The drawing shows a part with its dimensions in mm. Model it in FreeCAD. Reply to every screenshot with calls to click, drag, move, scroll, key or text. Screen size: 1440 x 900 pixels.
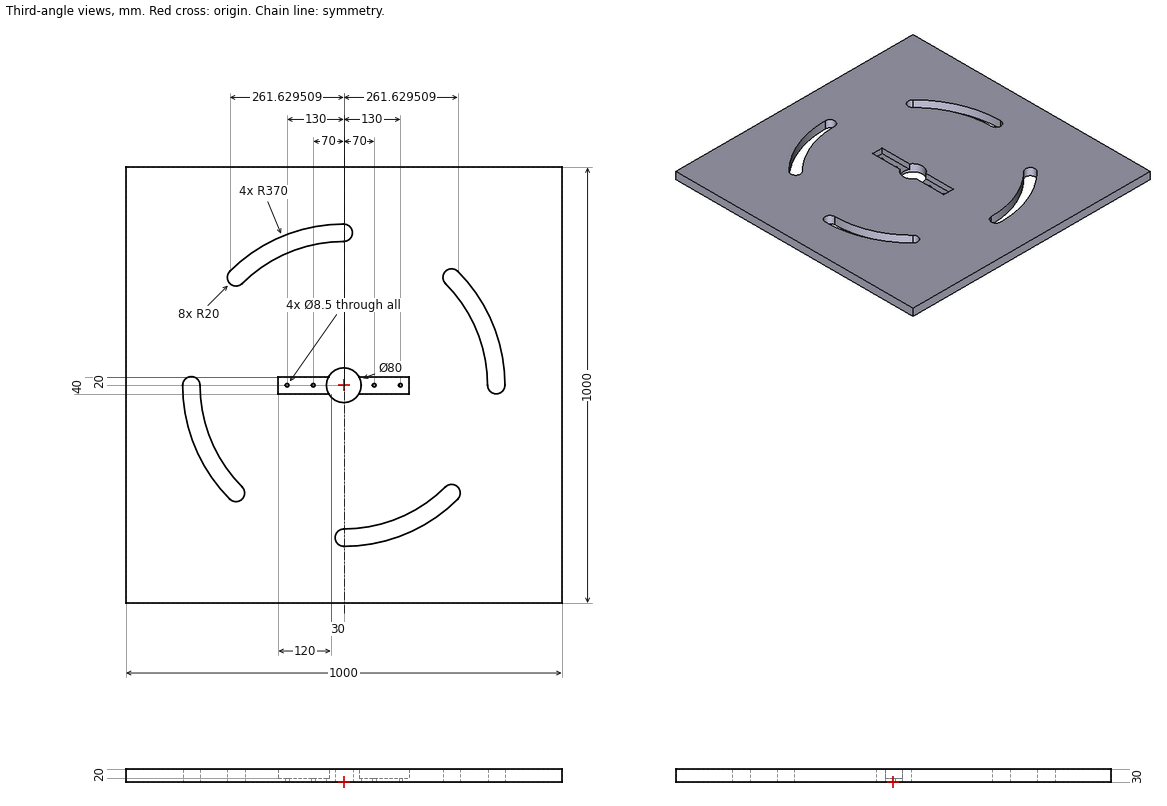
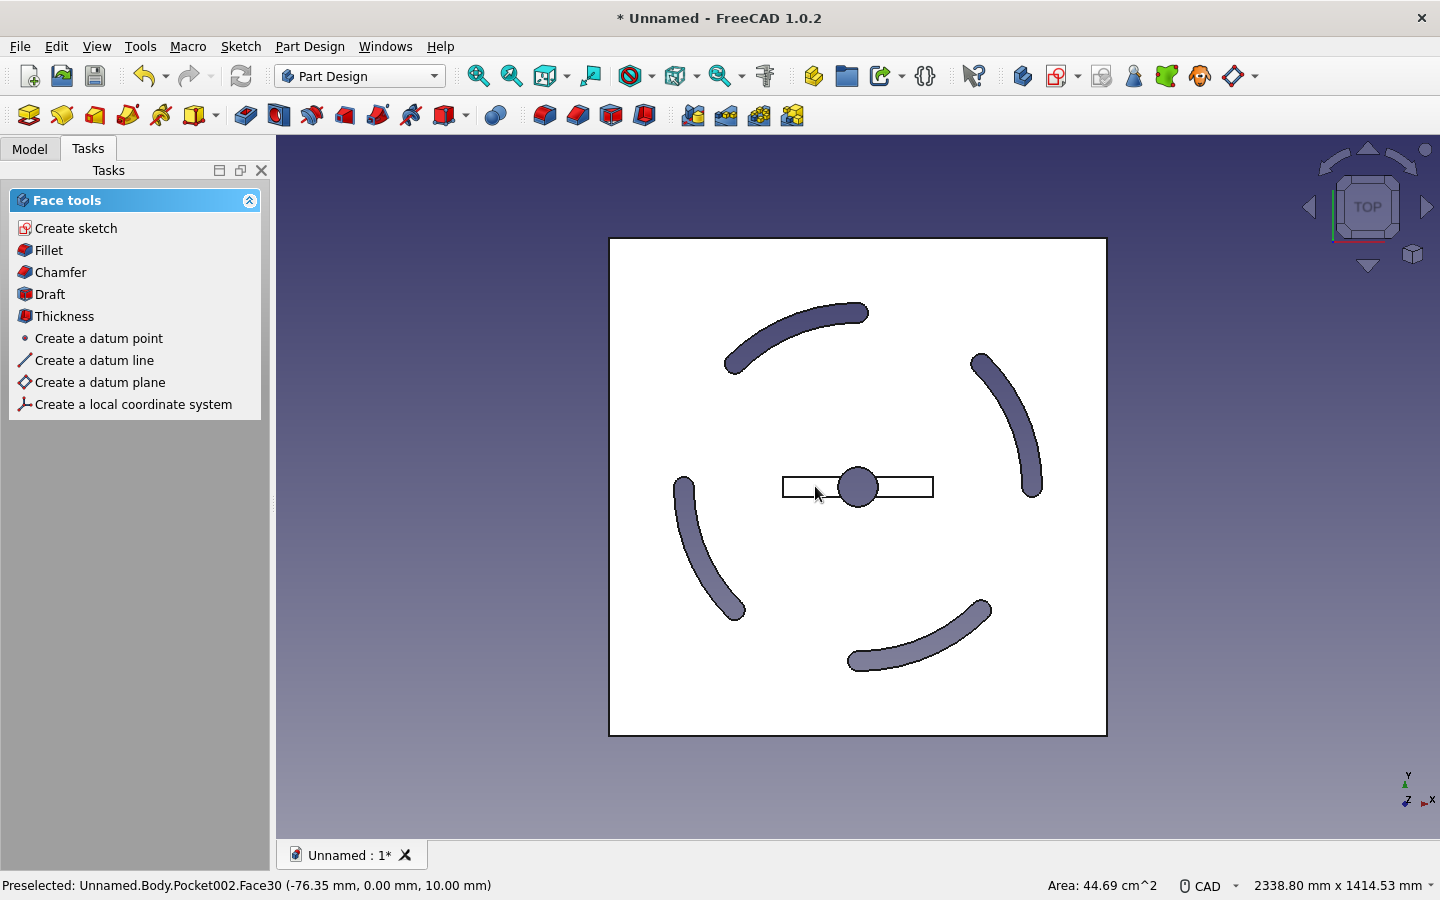
click(1056, 76)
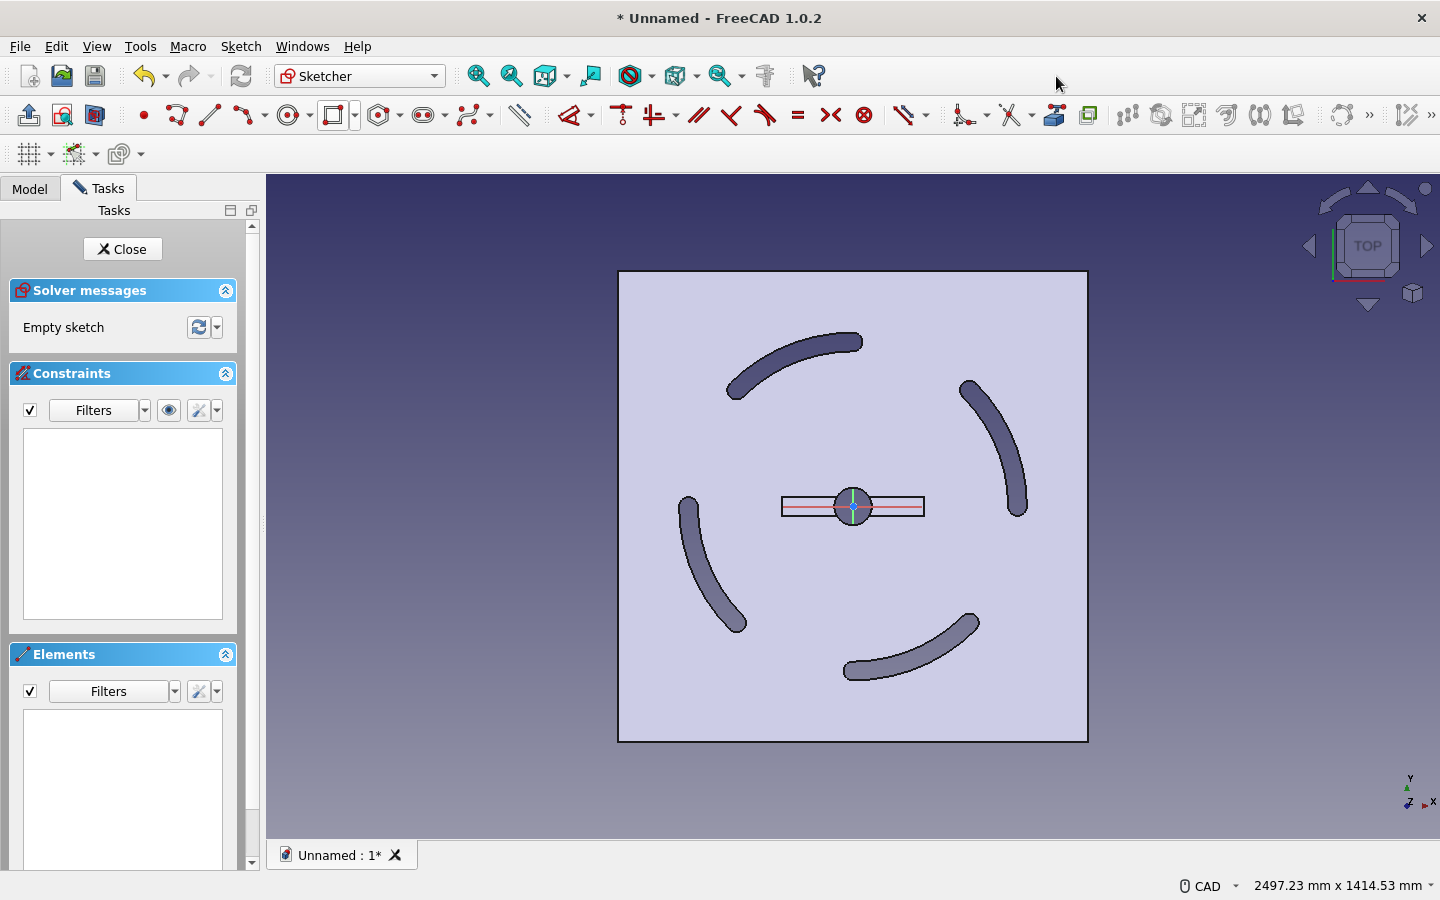
click(95, 116)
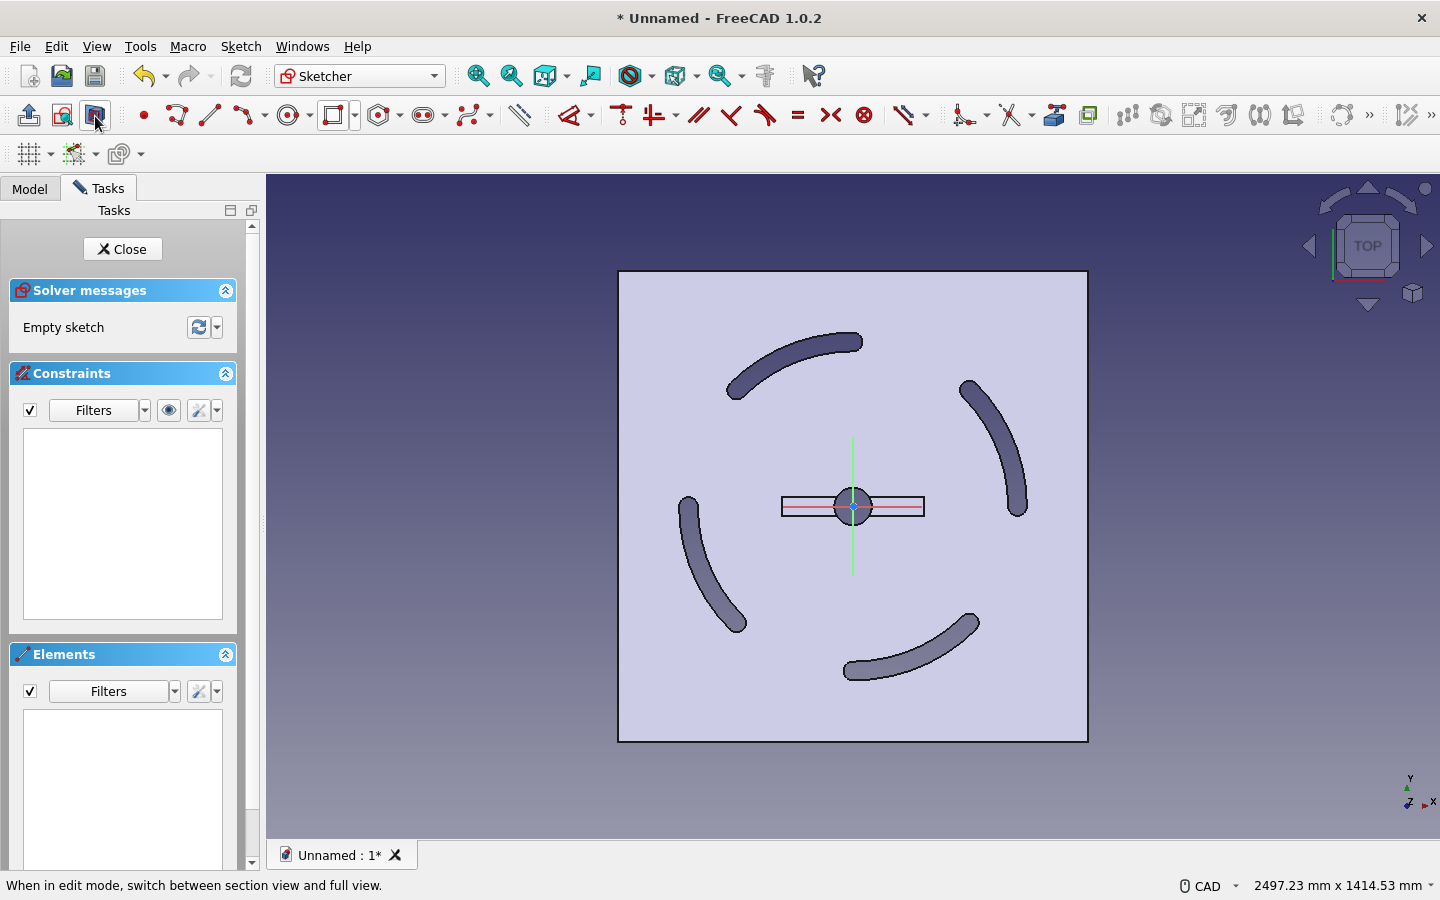
scroll(867, 506, up, 9)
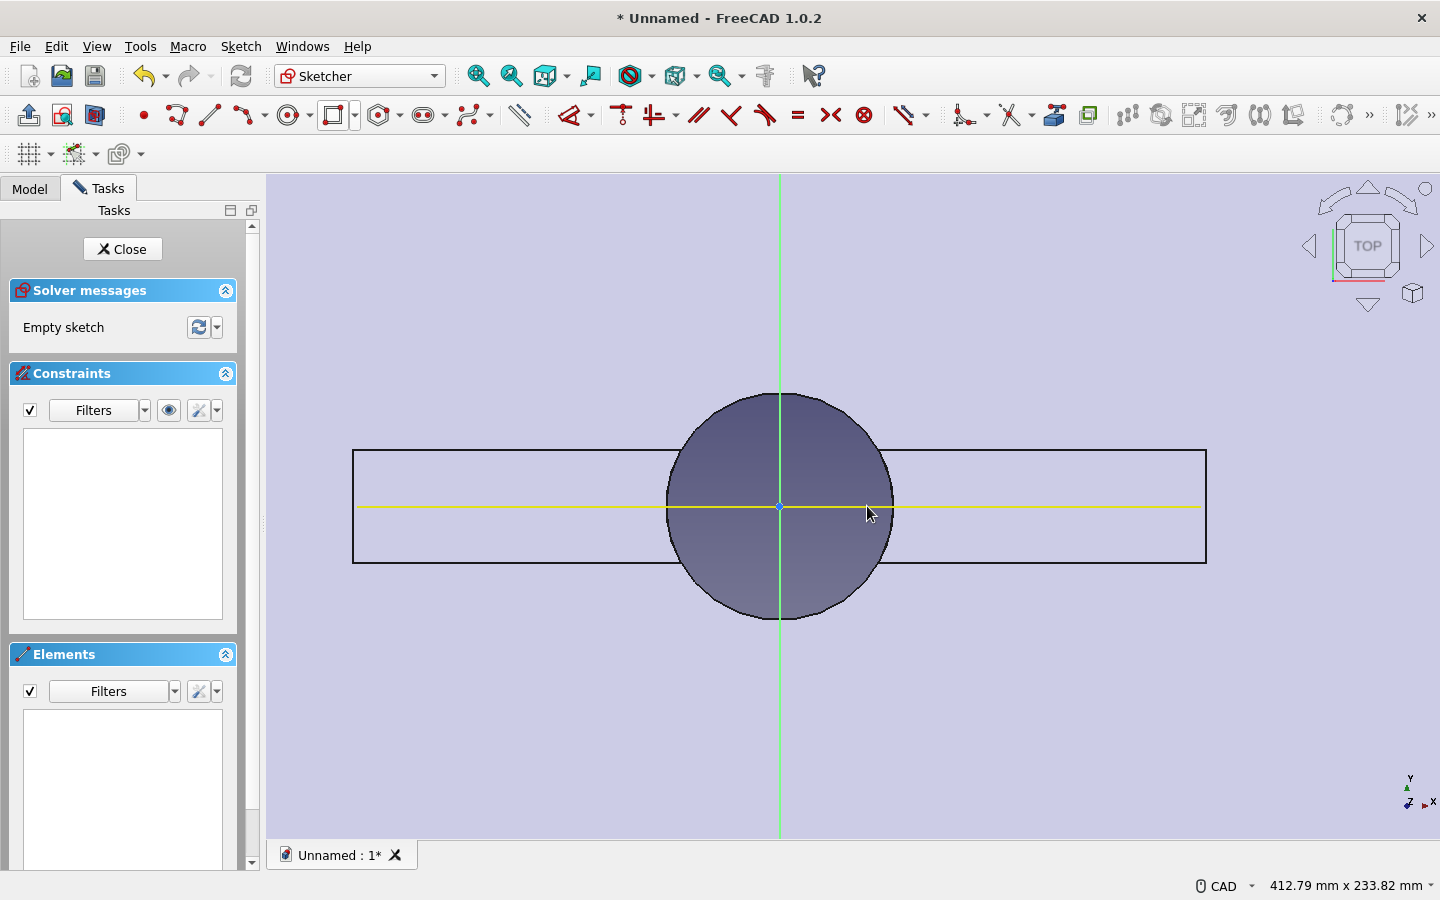
click(288, 116)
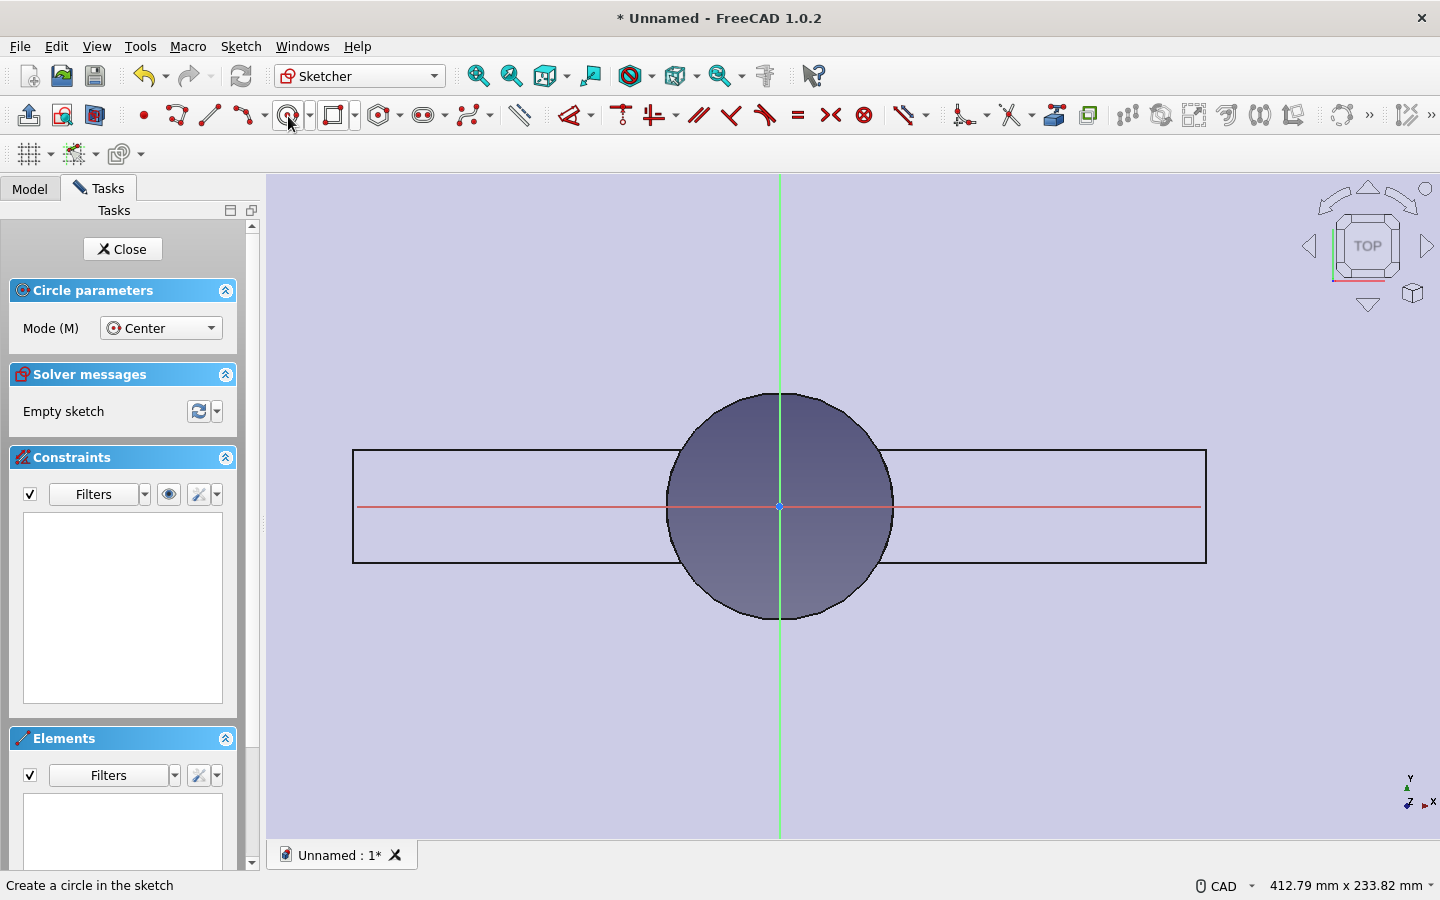
scroll(410, 506, up, 4)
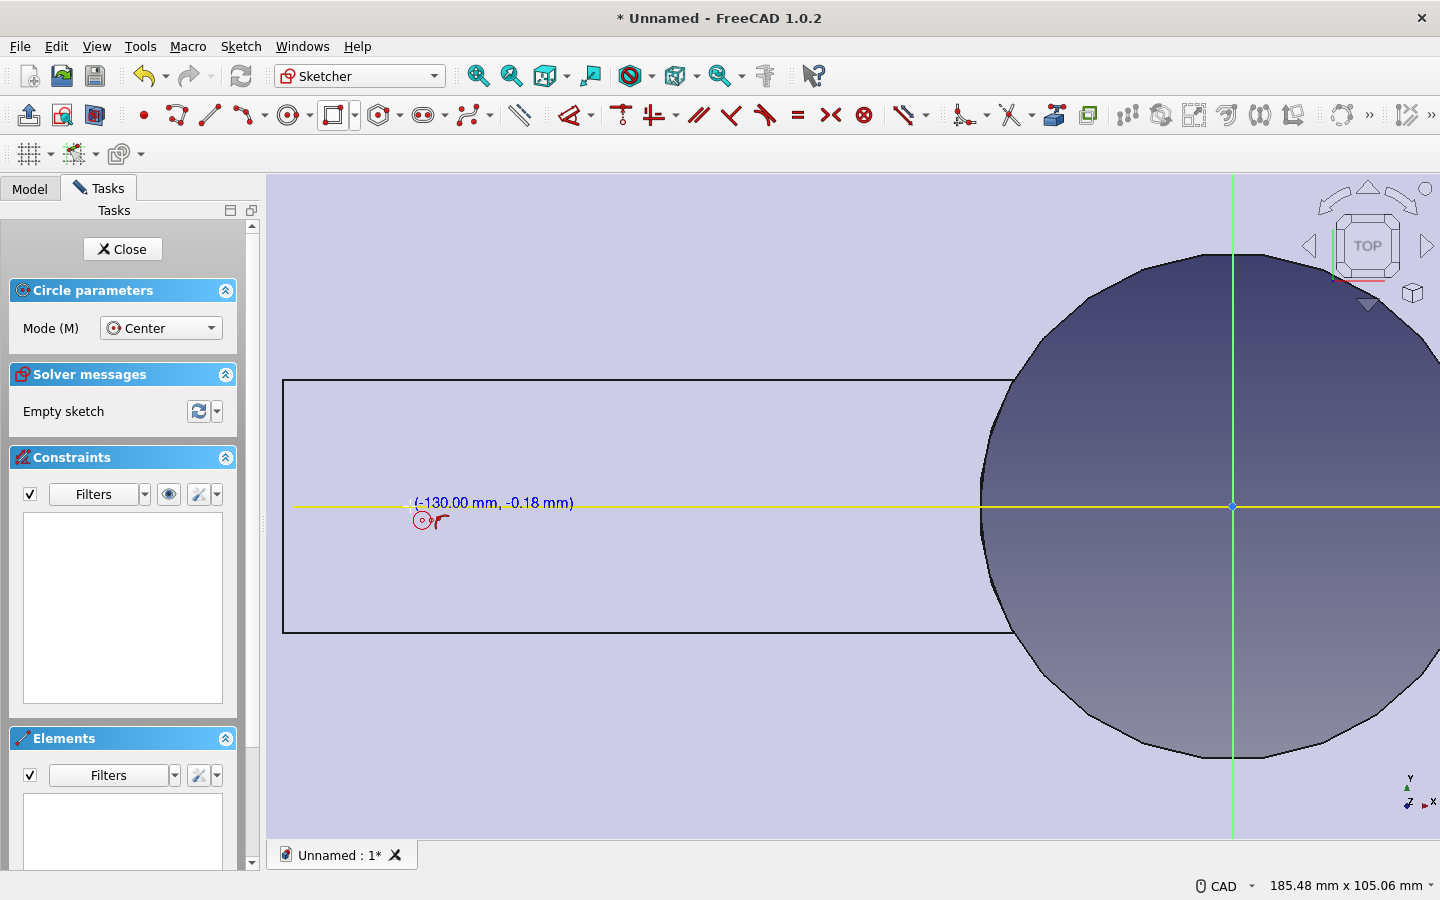
click(410, 506)
click(429, 487)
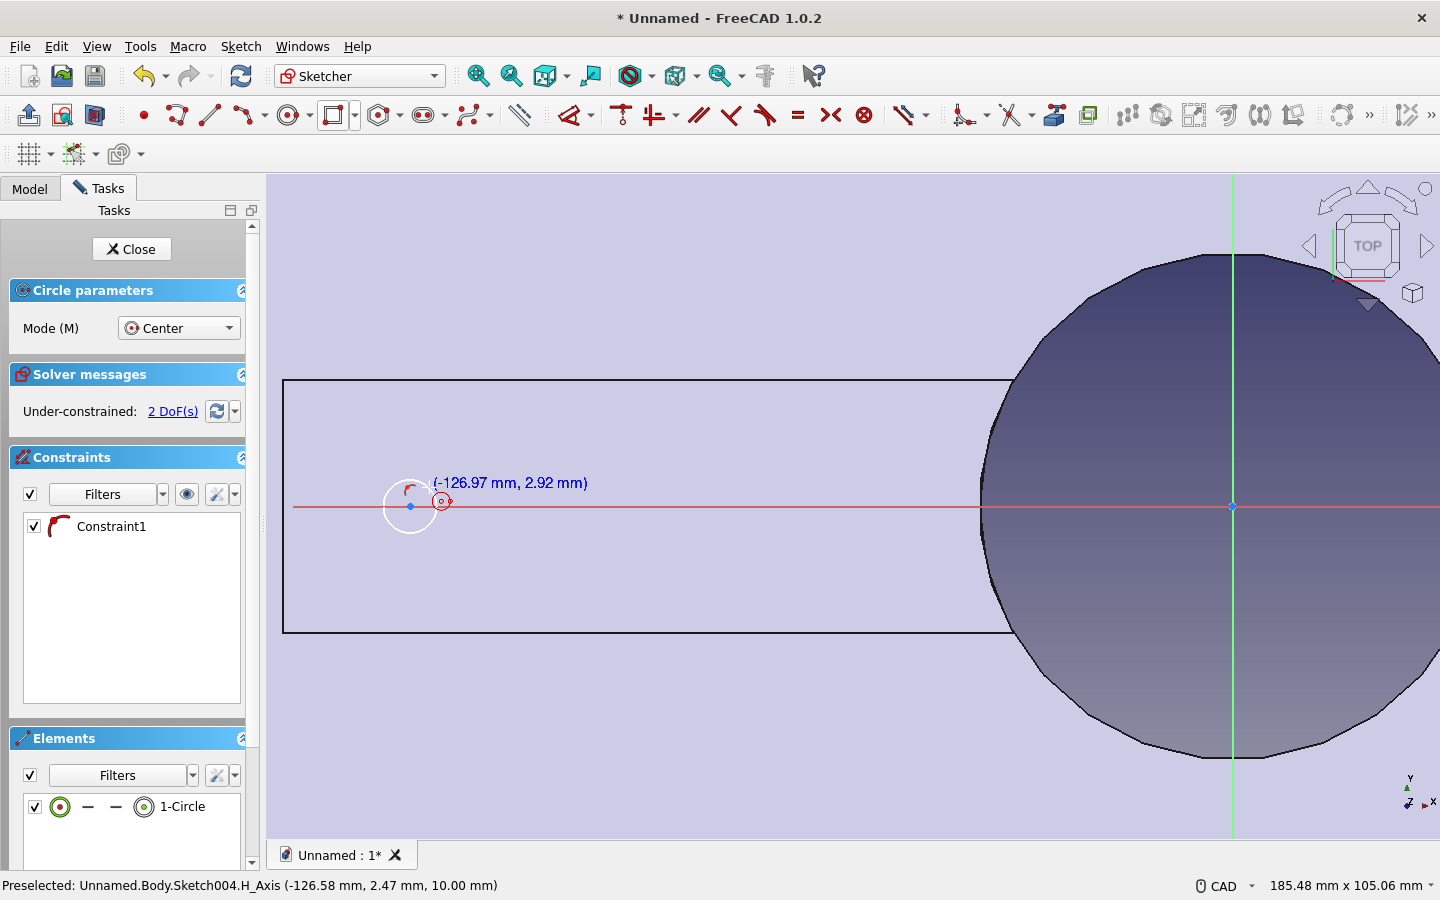
click(790, 506)
click(809, 487)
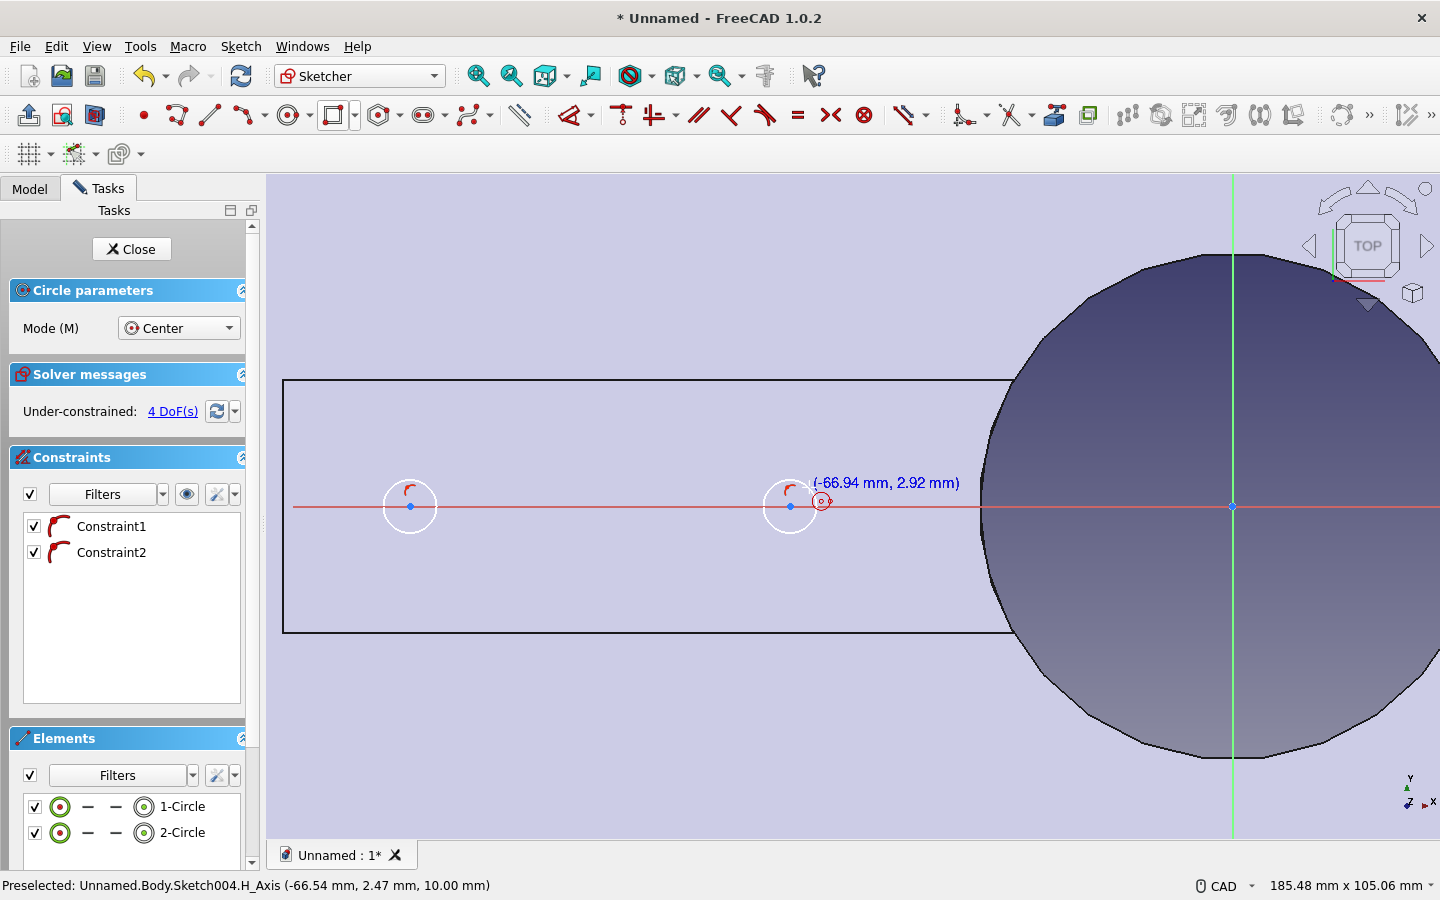
scroll(419, 506, down, 4)